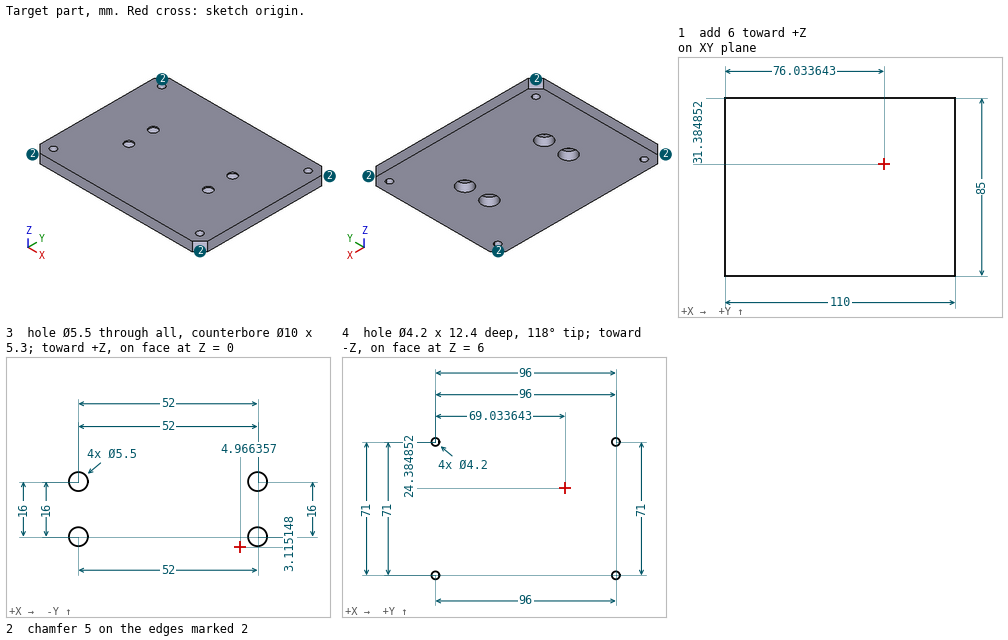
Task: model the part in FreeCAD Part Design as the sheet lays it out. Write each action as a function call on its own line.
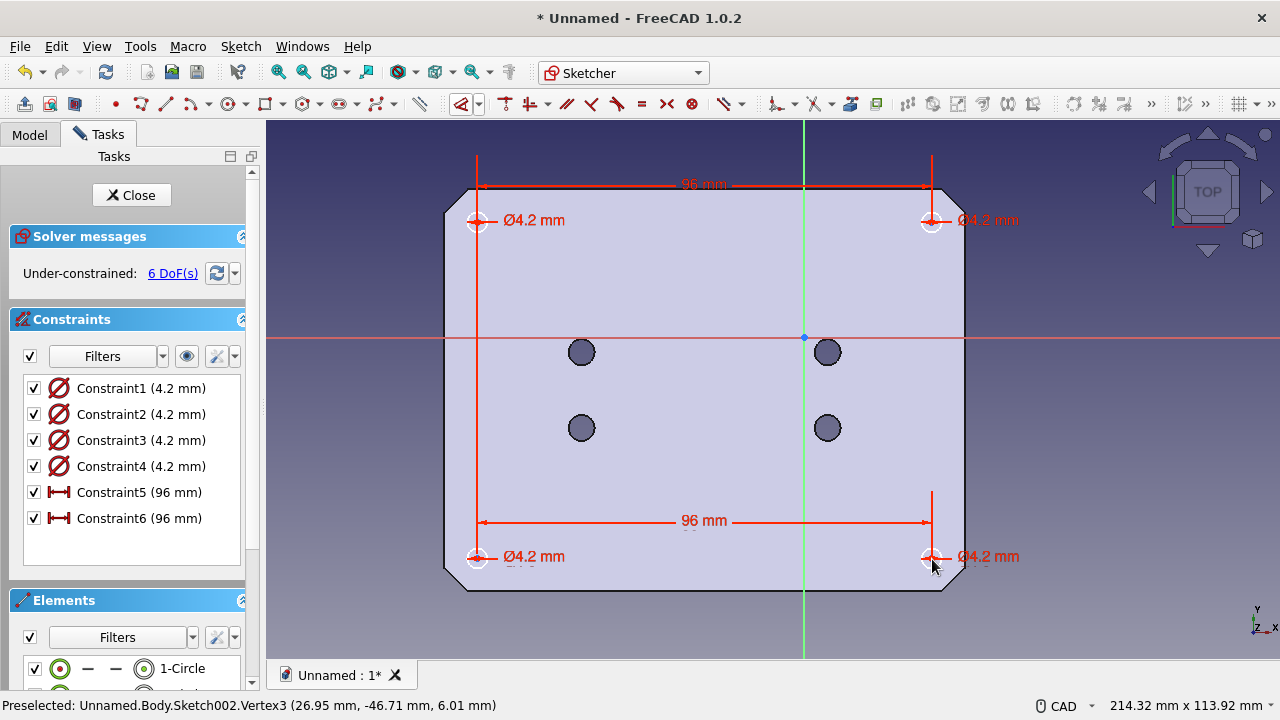
click(932, 222)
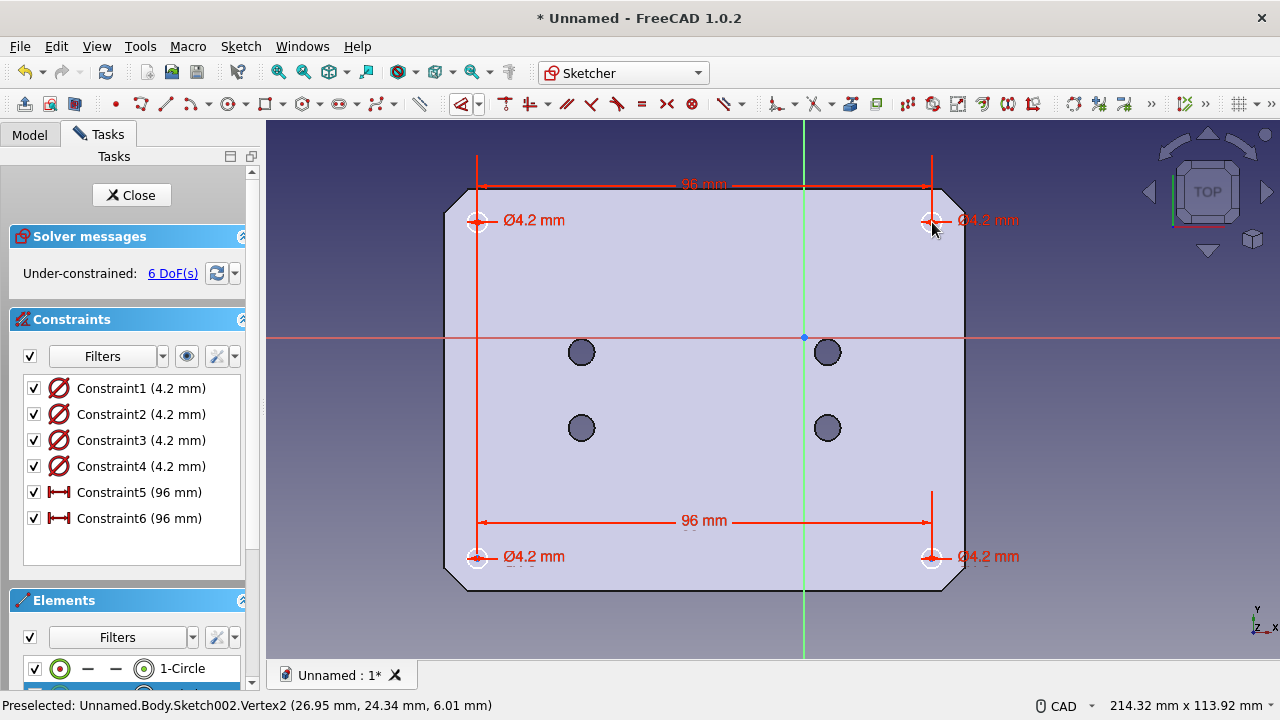
click(932, 559)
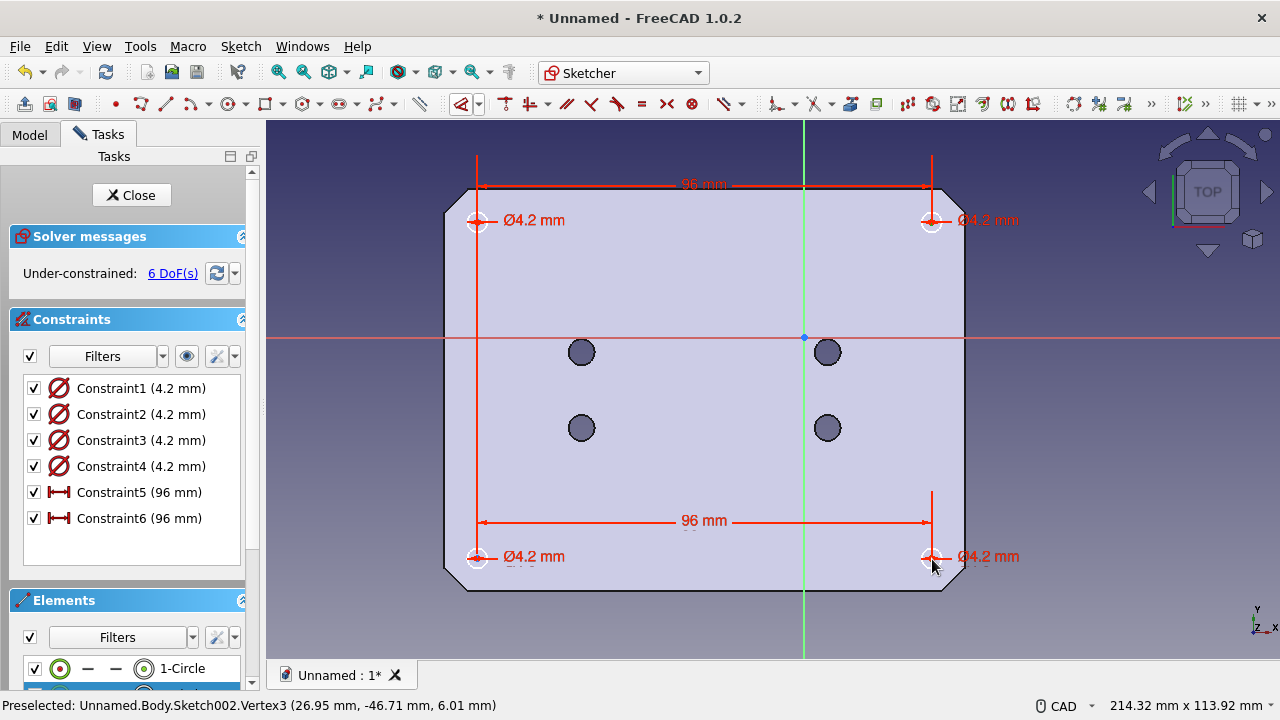
key(i)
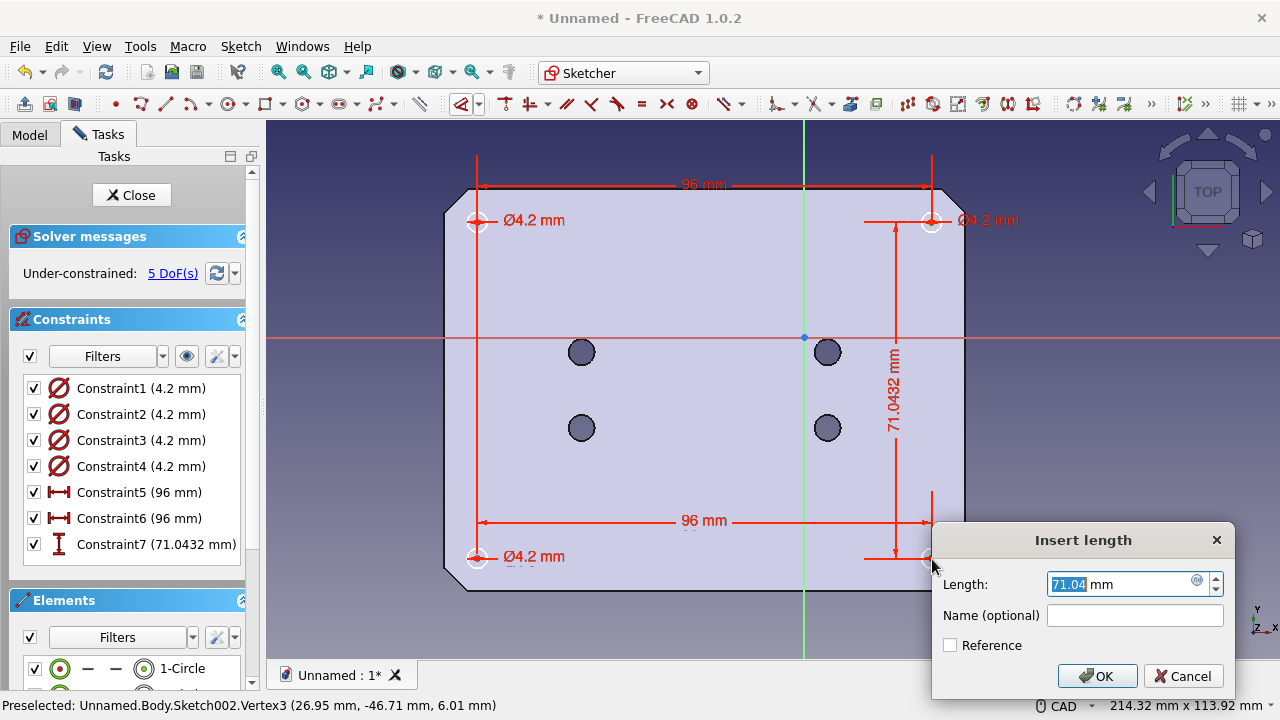
text(71)
key(Return)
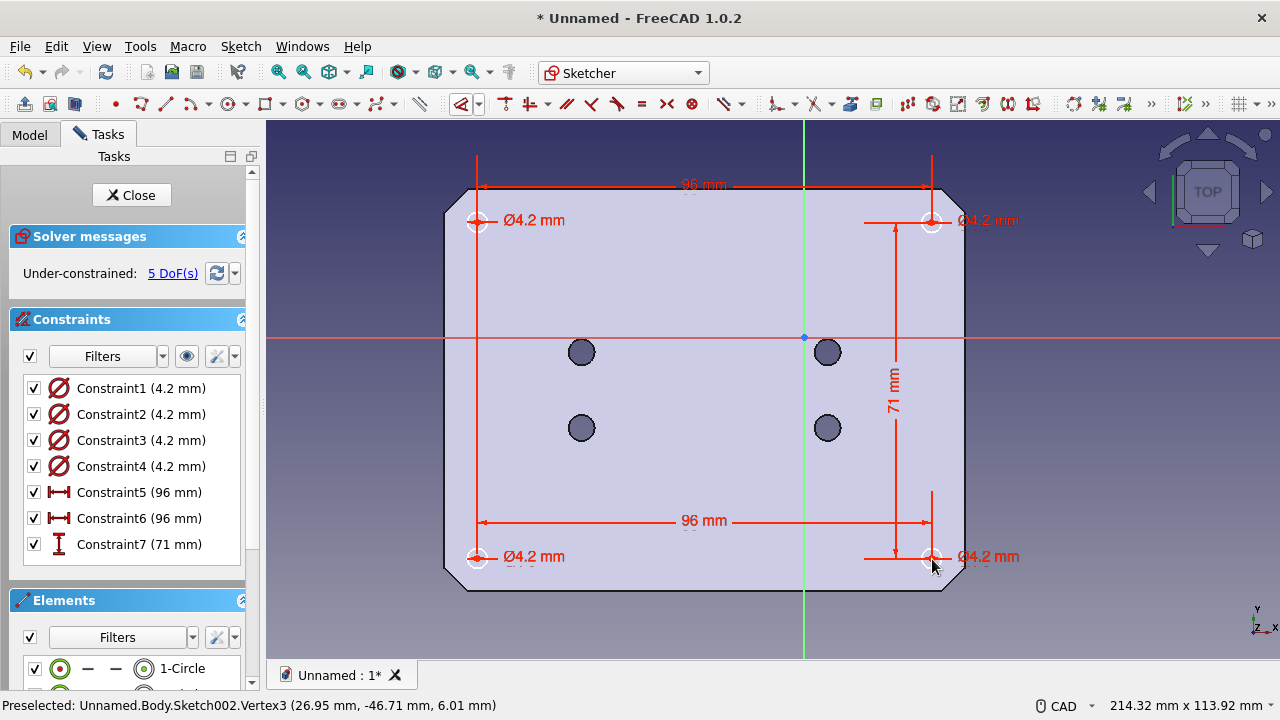
click(477, 222)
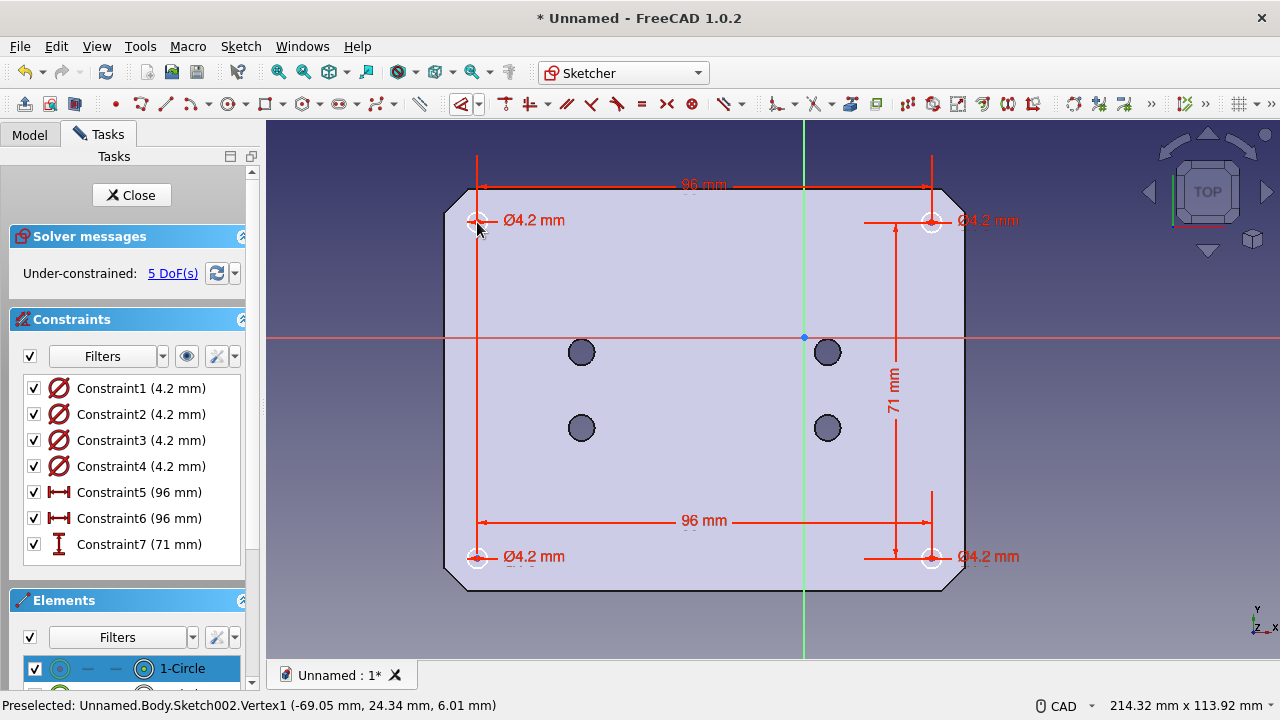
click(932, 559)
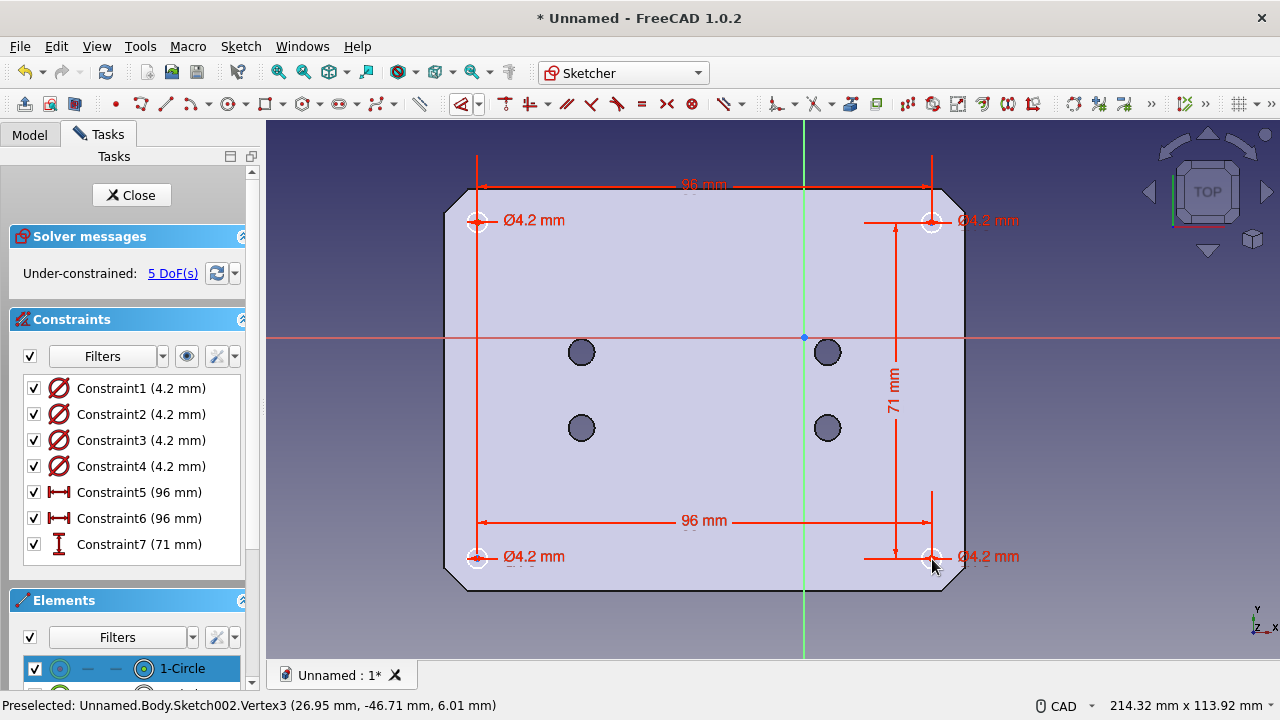
key(i)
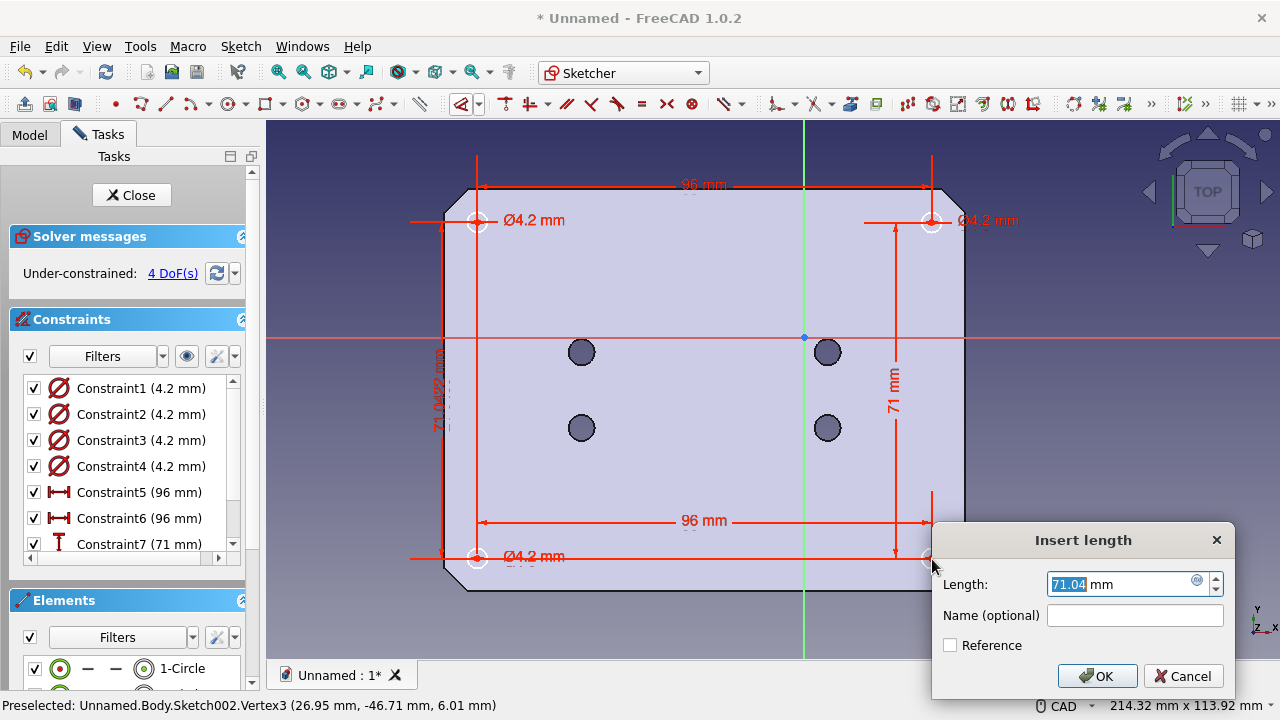
text(71)
key(Return)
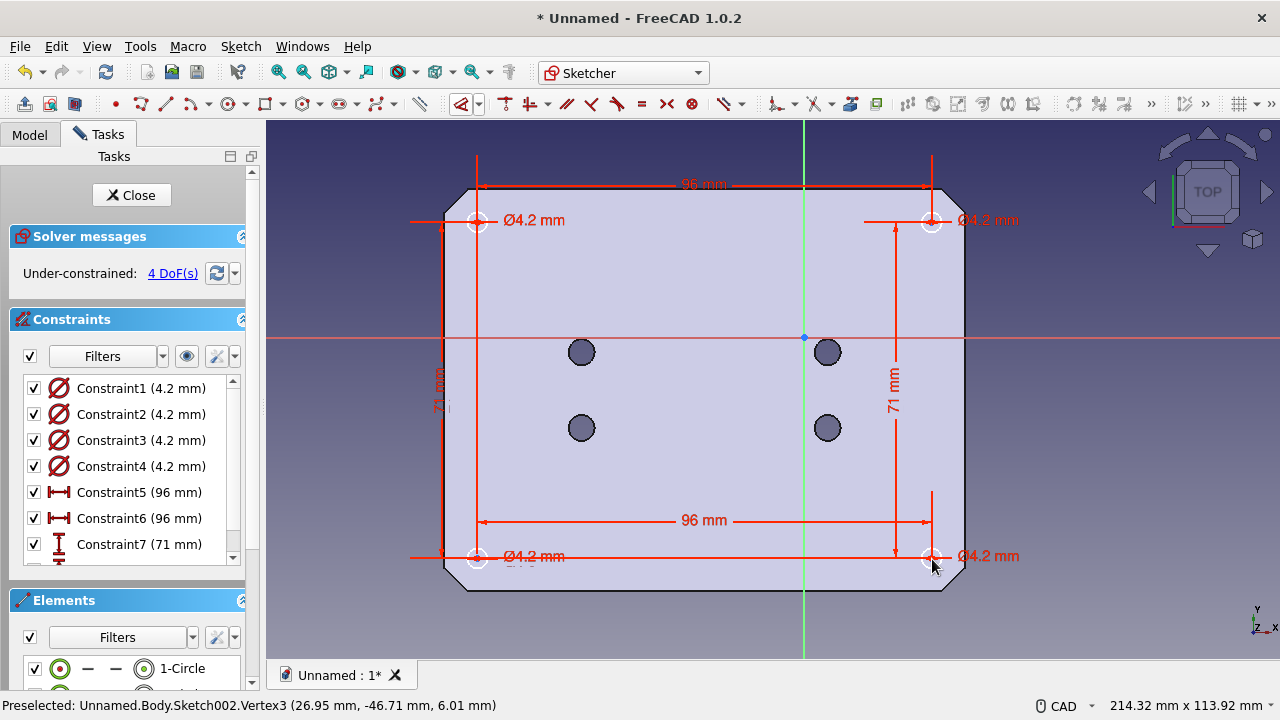
click(932, 558)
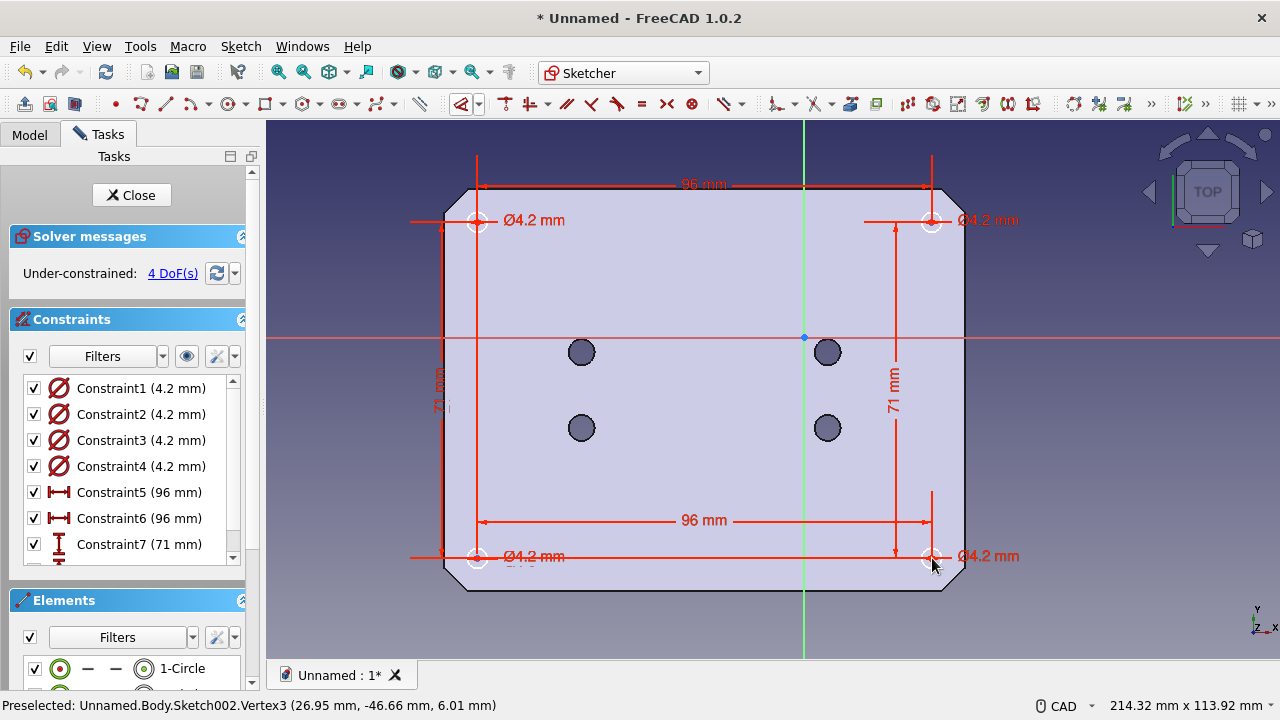
click(477, 559)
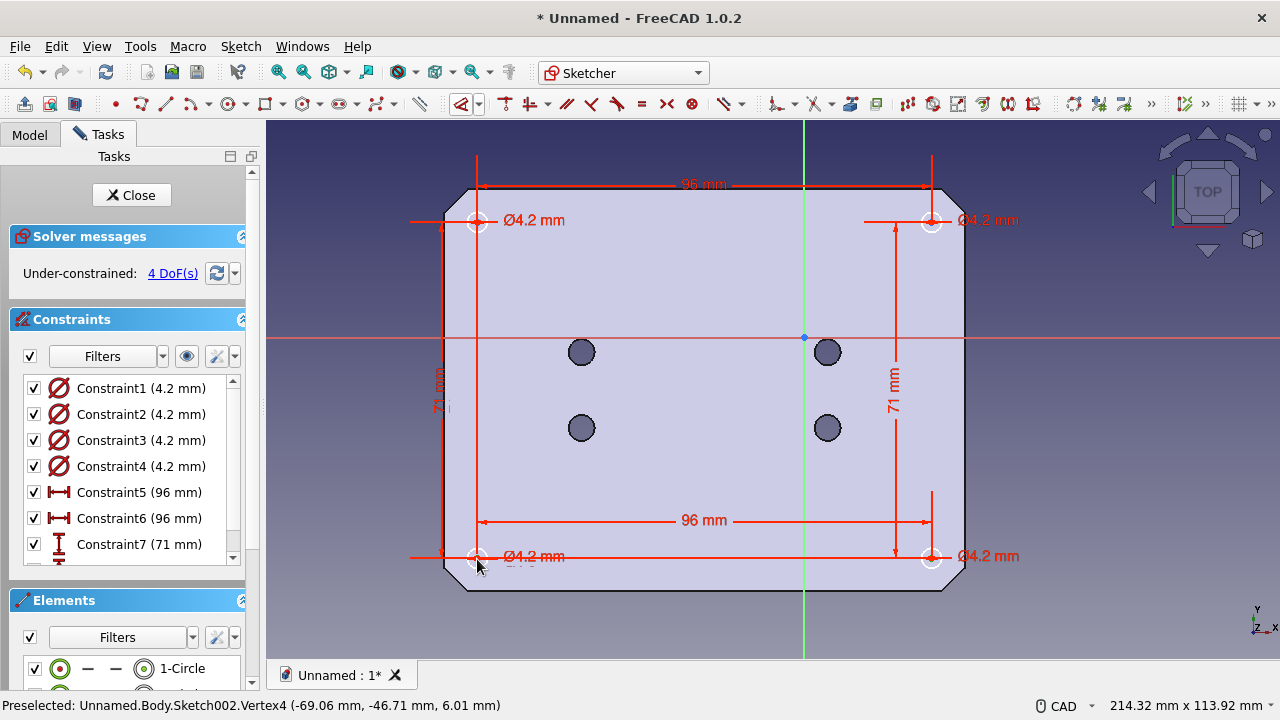
key(l)